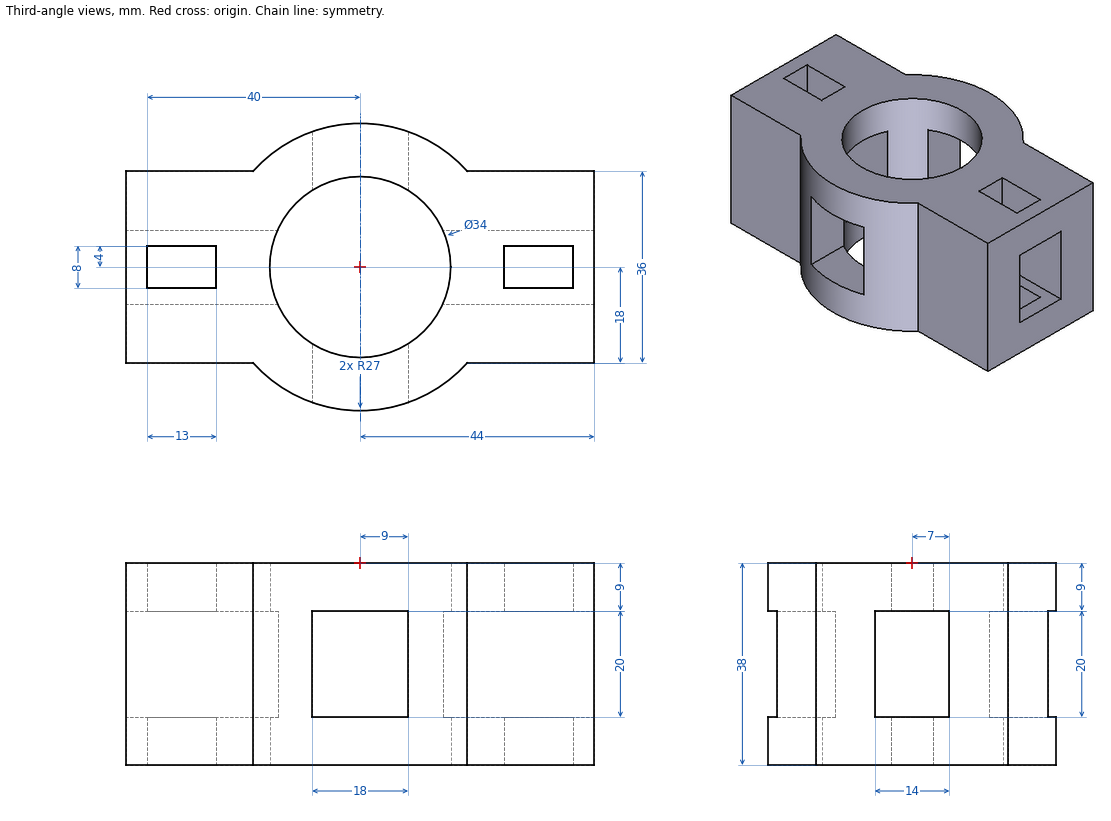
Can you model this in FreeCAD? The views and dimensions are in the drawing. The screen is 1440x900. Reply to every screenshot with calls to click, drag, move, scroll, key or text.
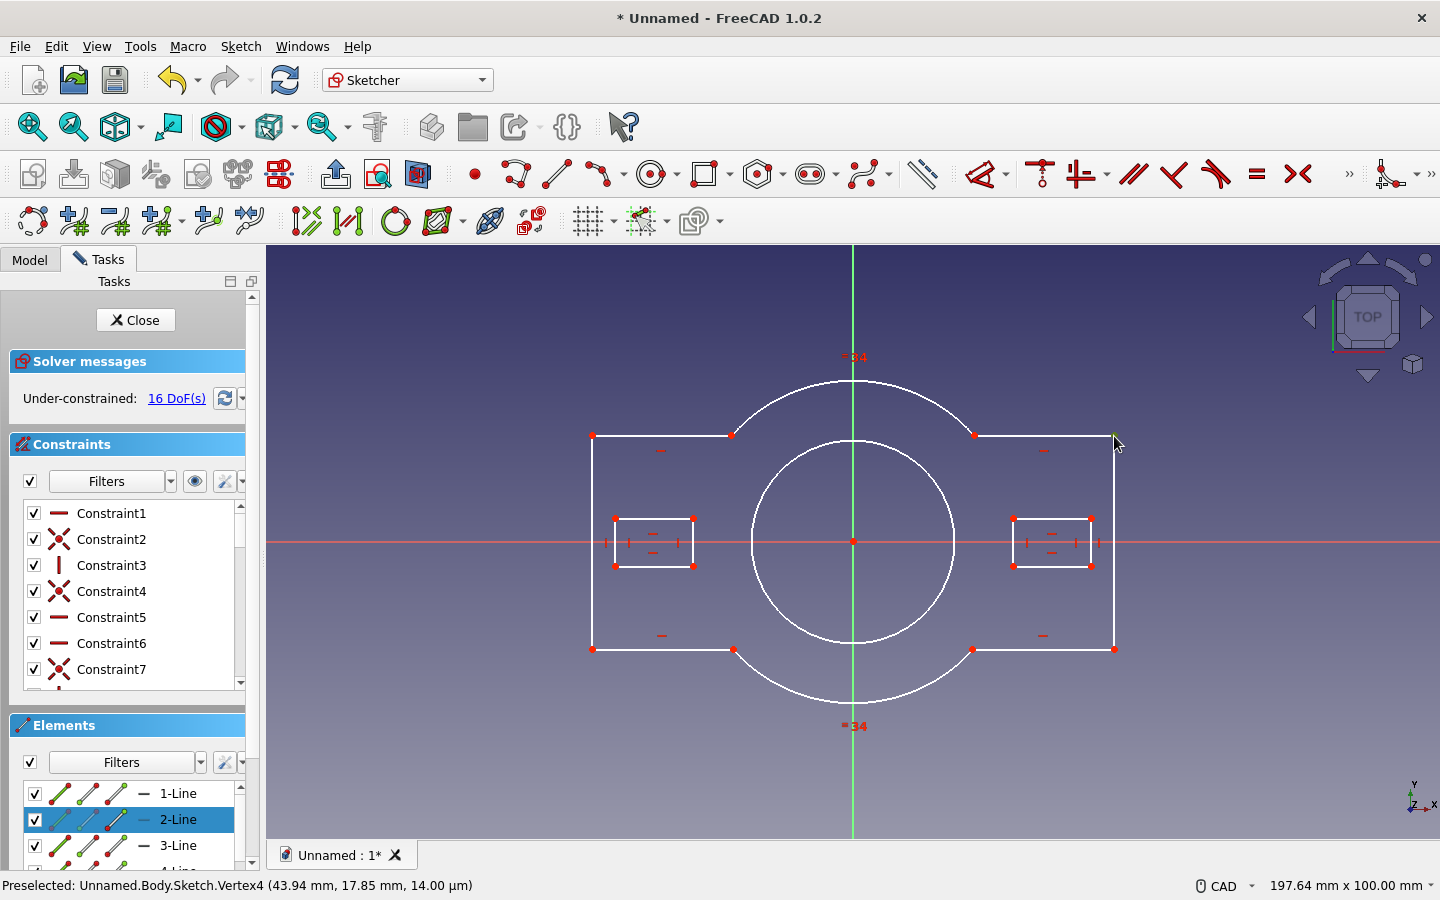
click(592, 436)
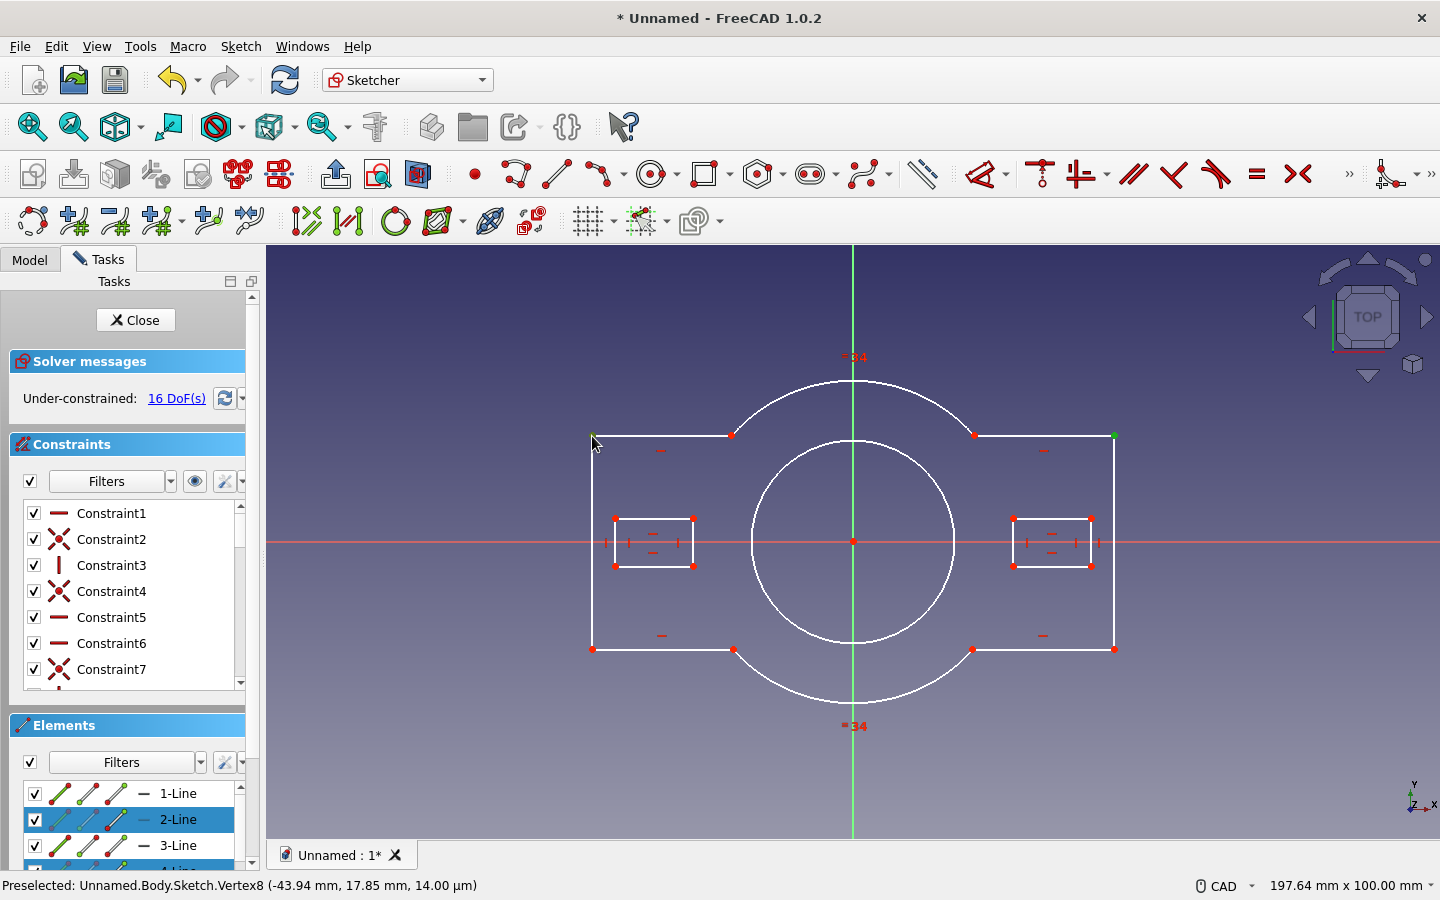
click(853, 773)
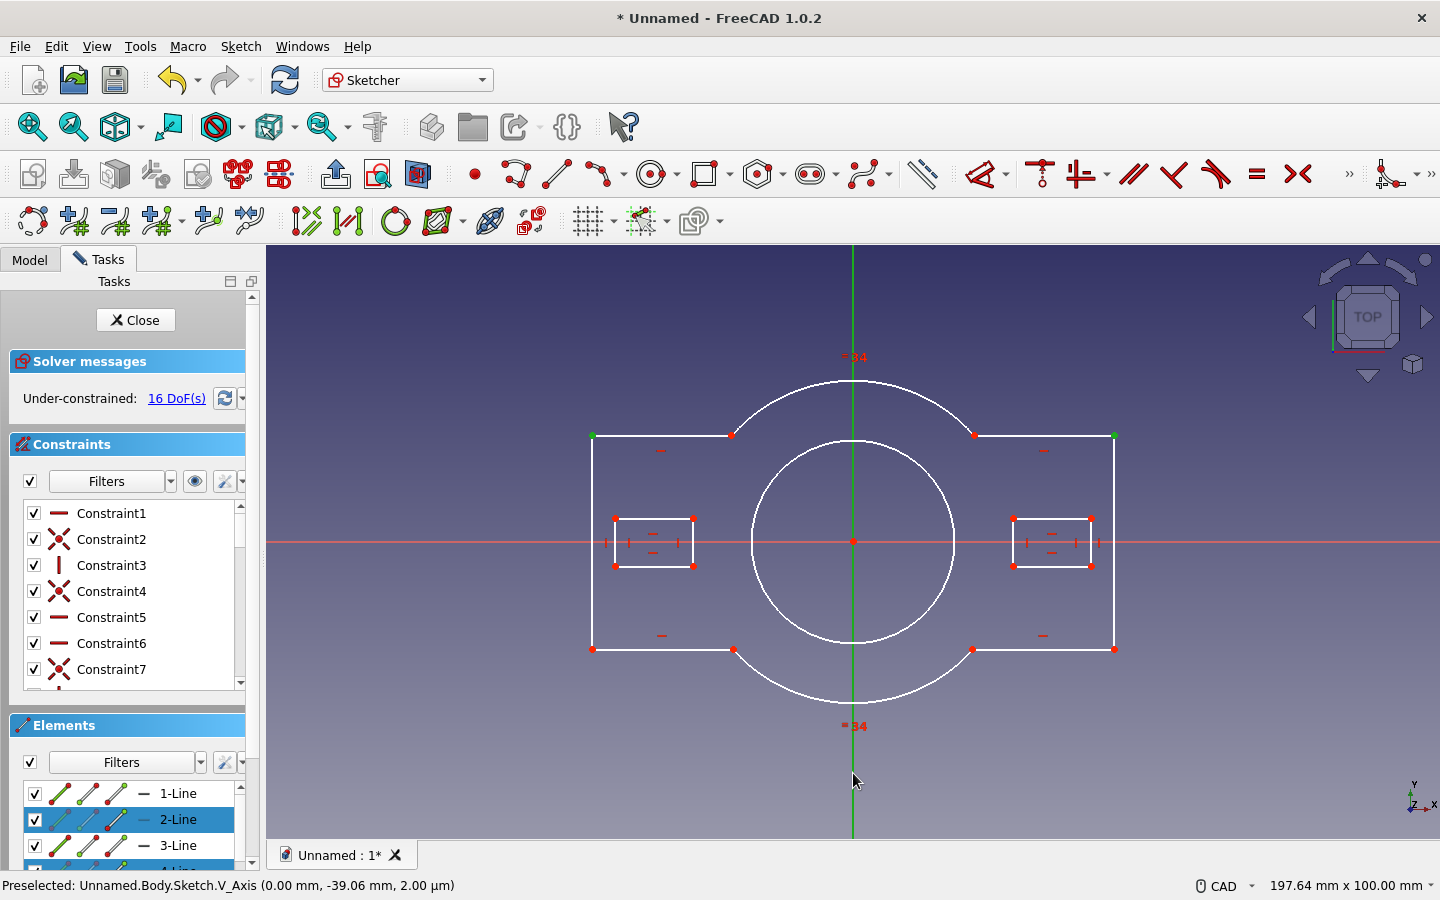
click(1298, 174)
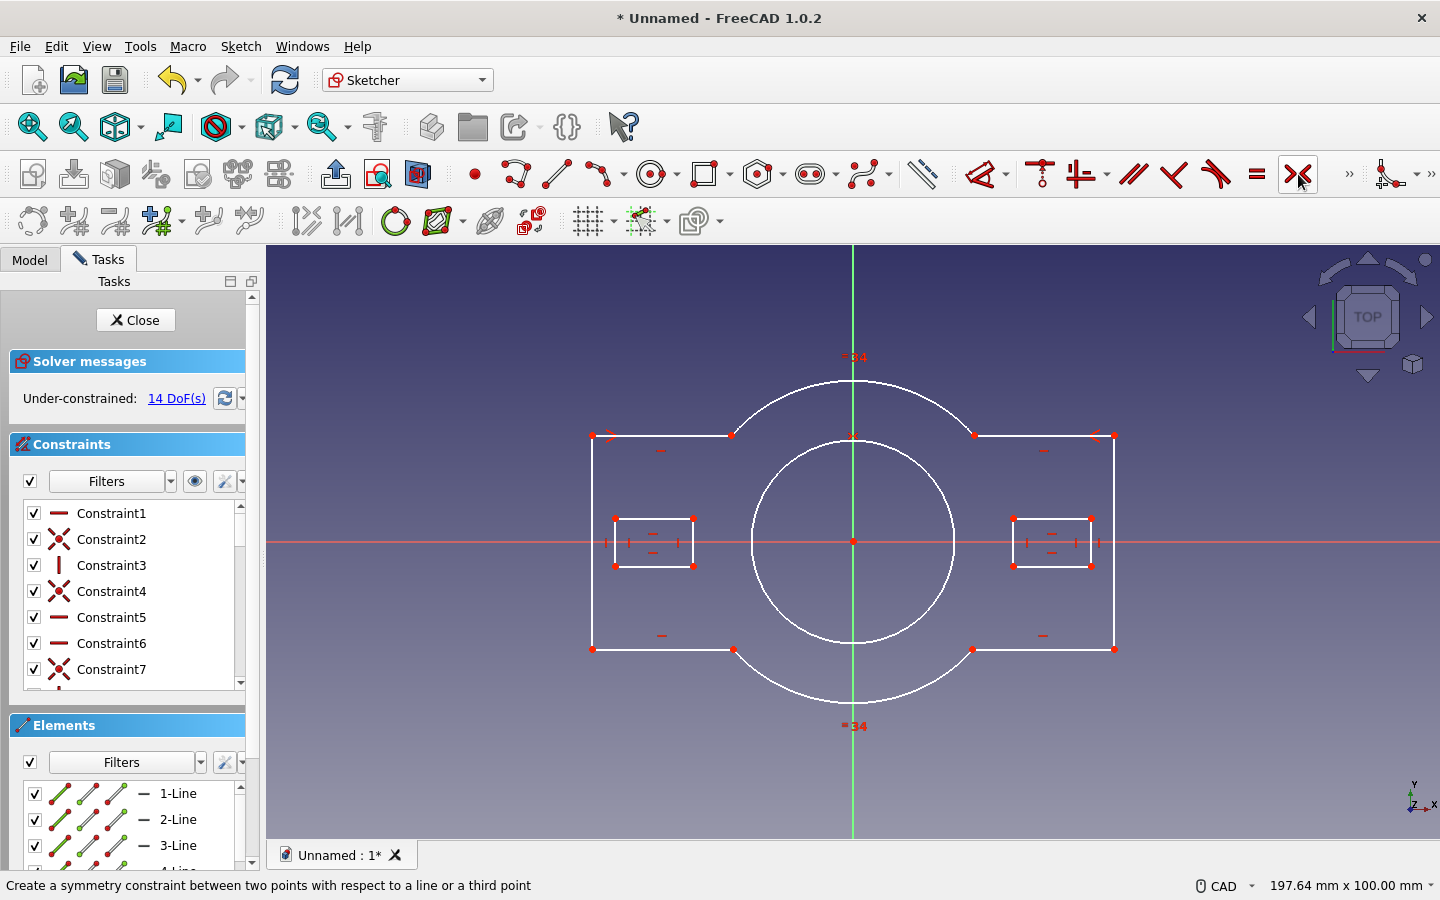
click(693, 519)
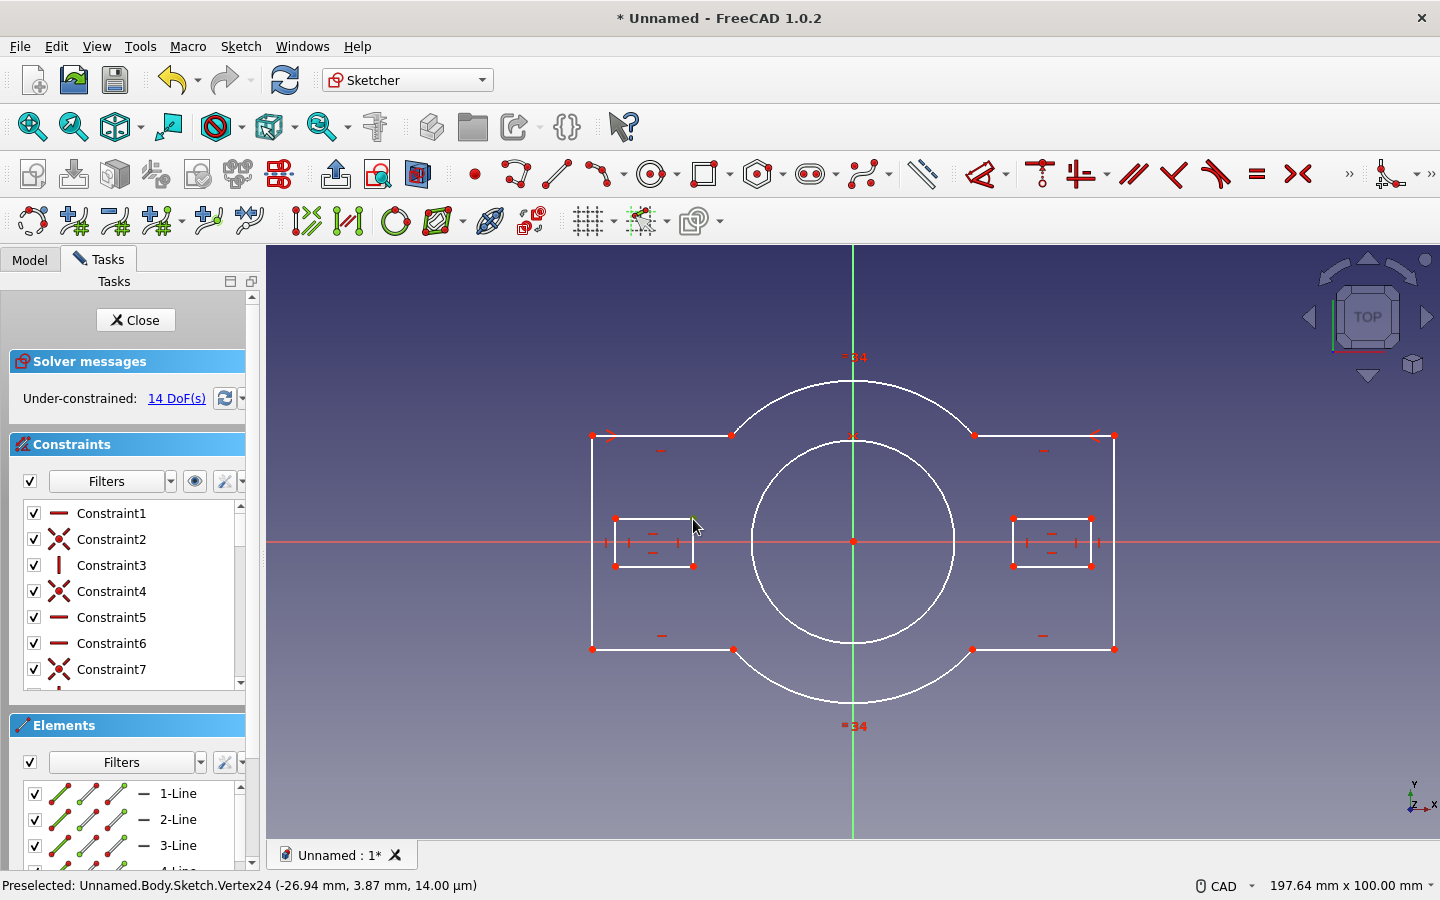
click(1013, 519)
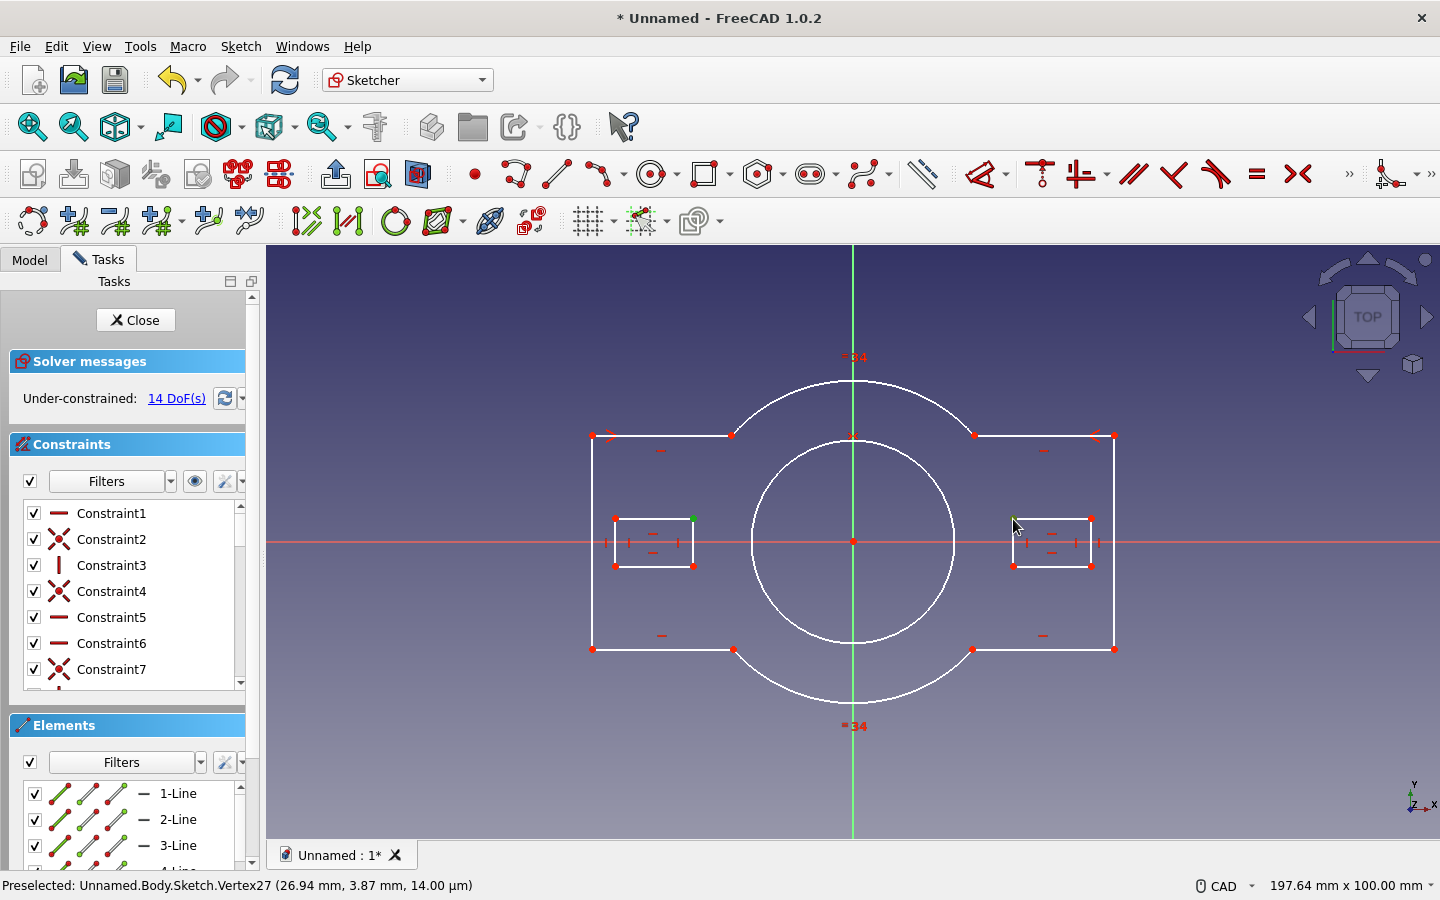
click(853, 773)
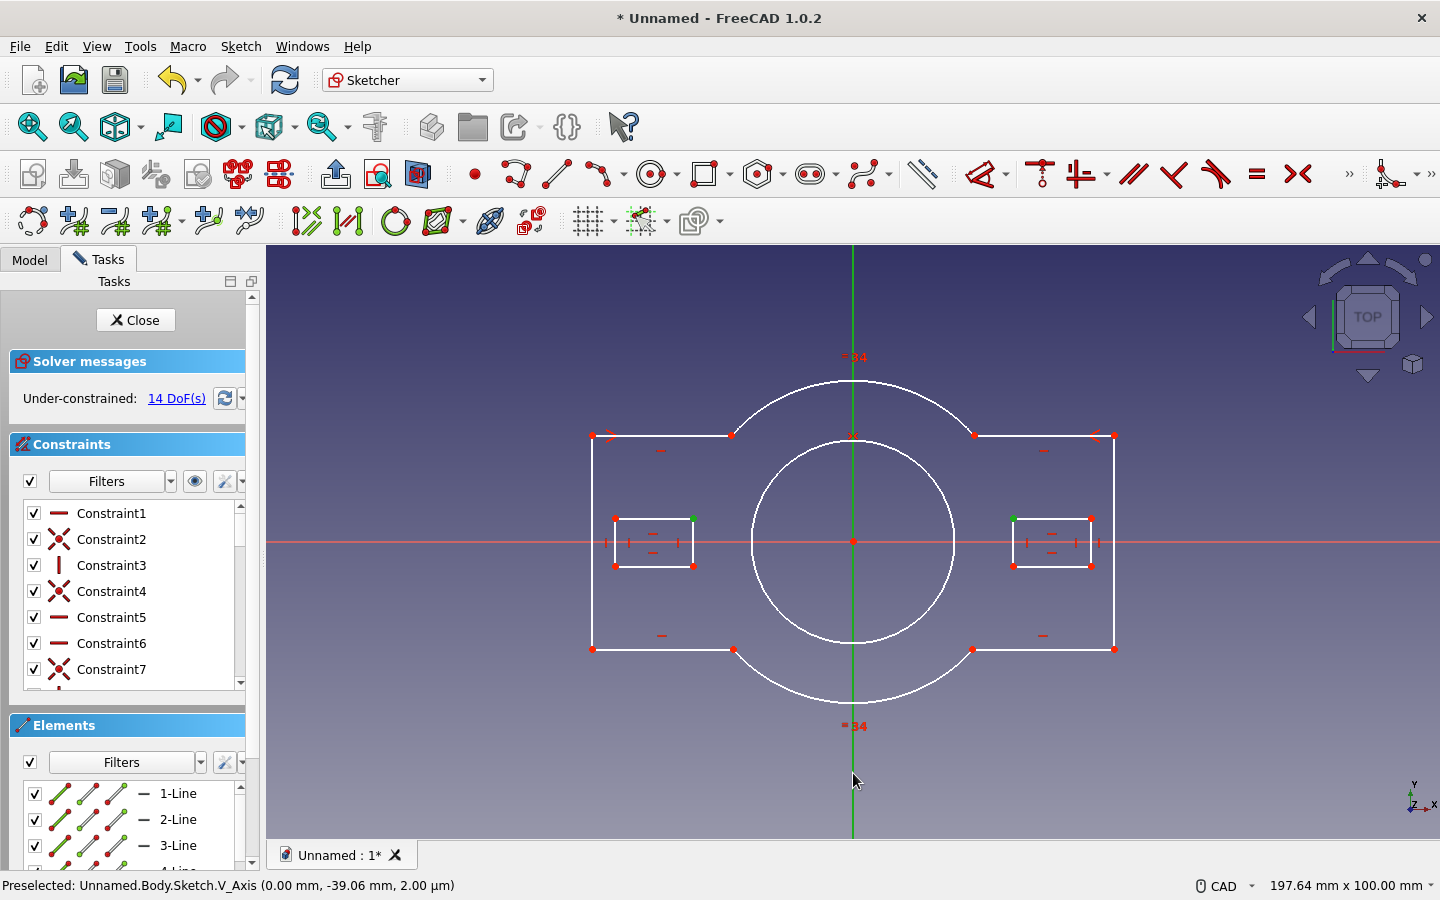
click(1298, 174)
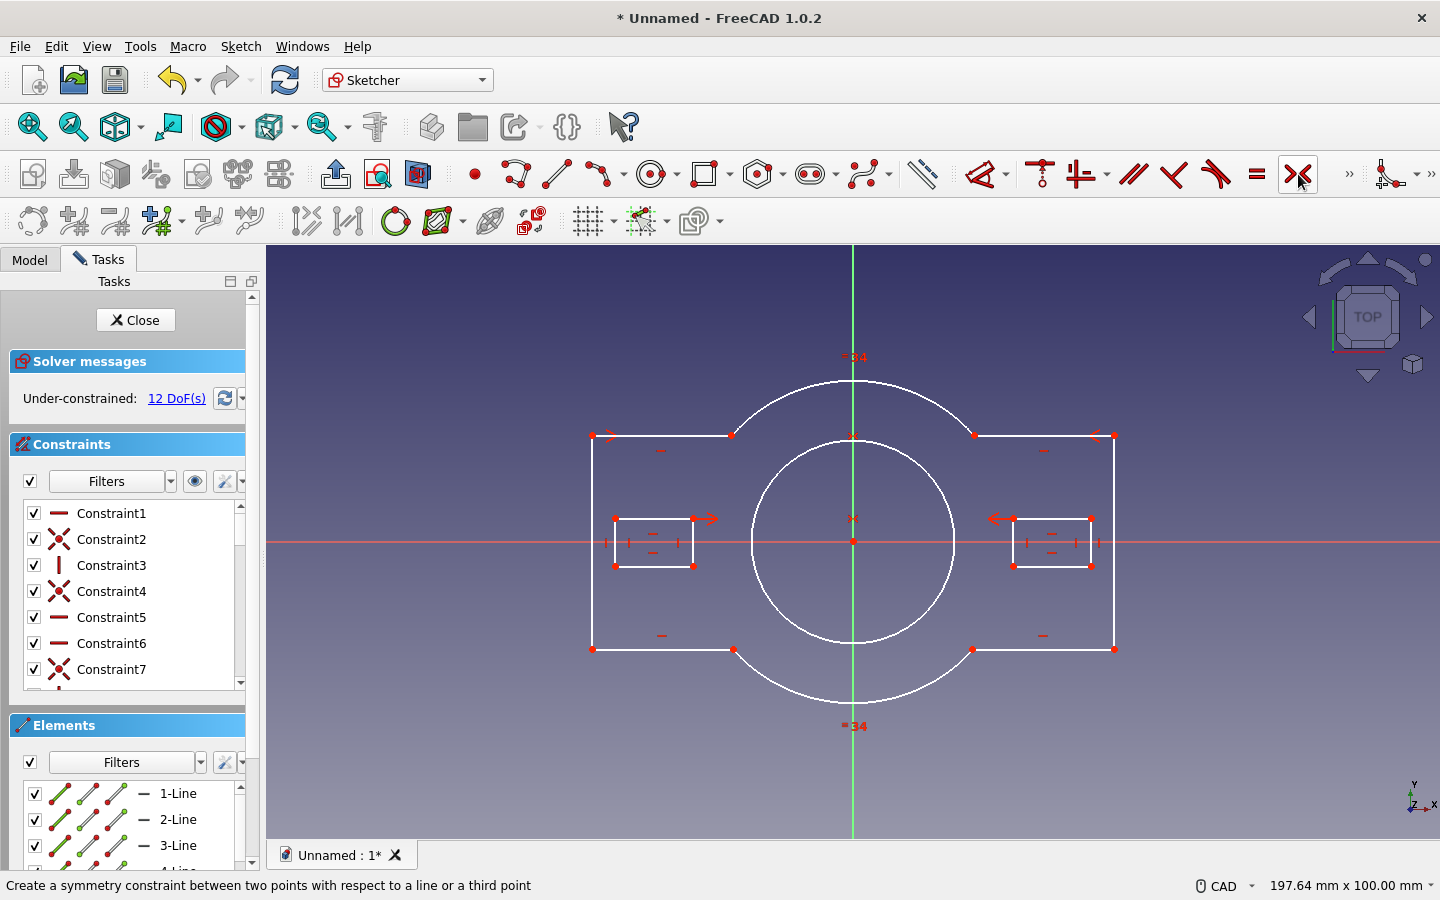
click(615, 567)